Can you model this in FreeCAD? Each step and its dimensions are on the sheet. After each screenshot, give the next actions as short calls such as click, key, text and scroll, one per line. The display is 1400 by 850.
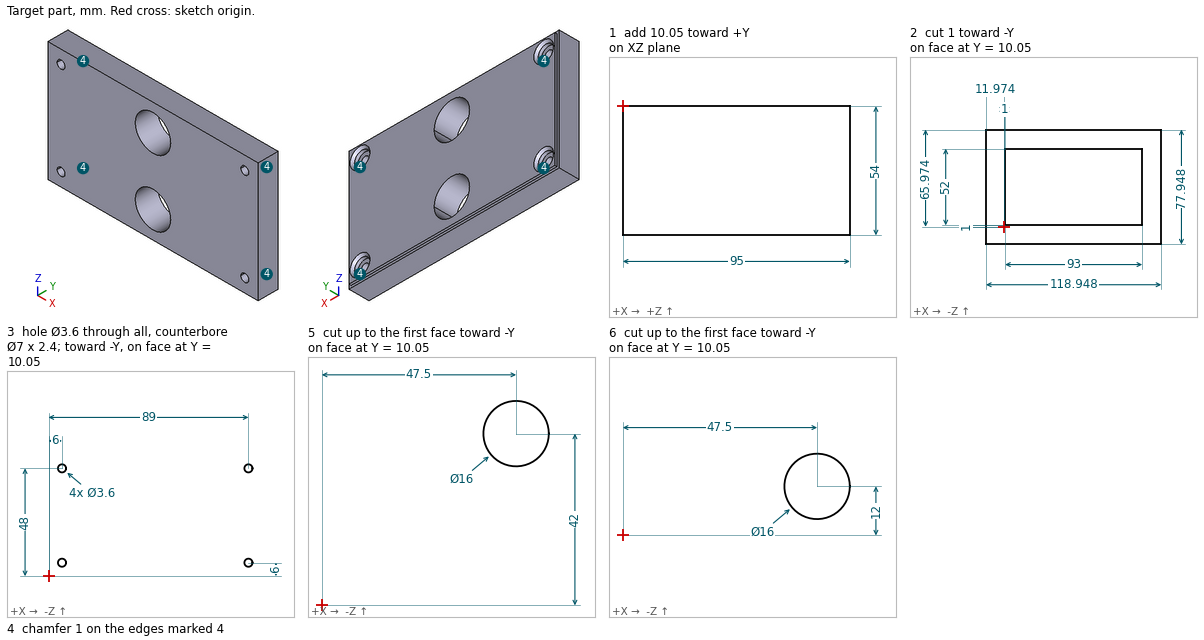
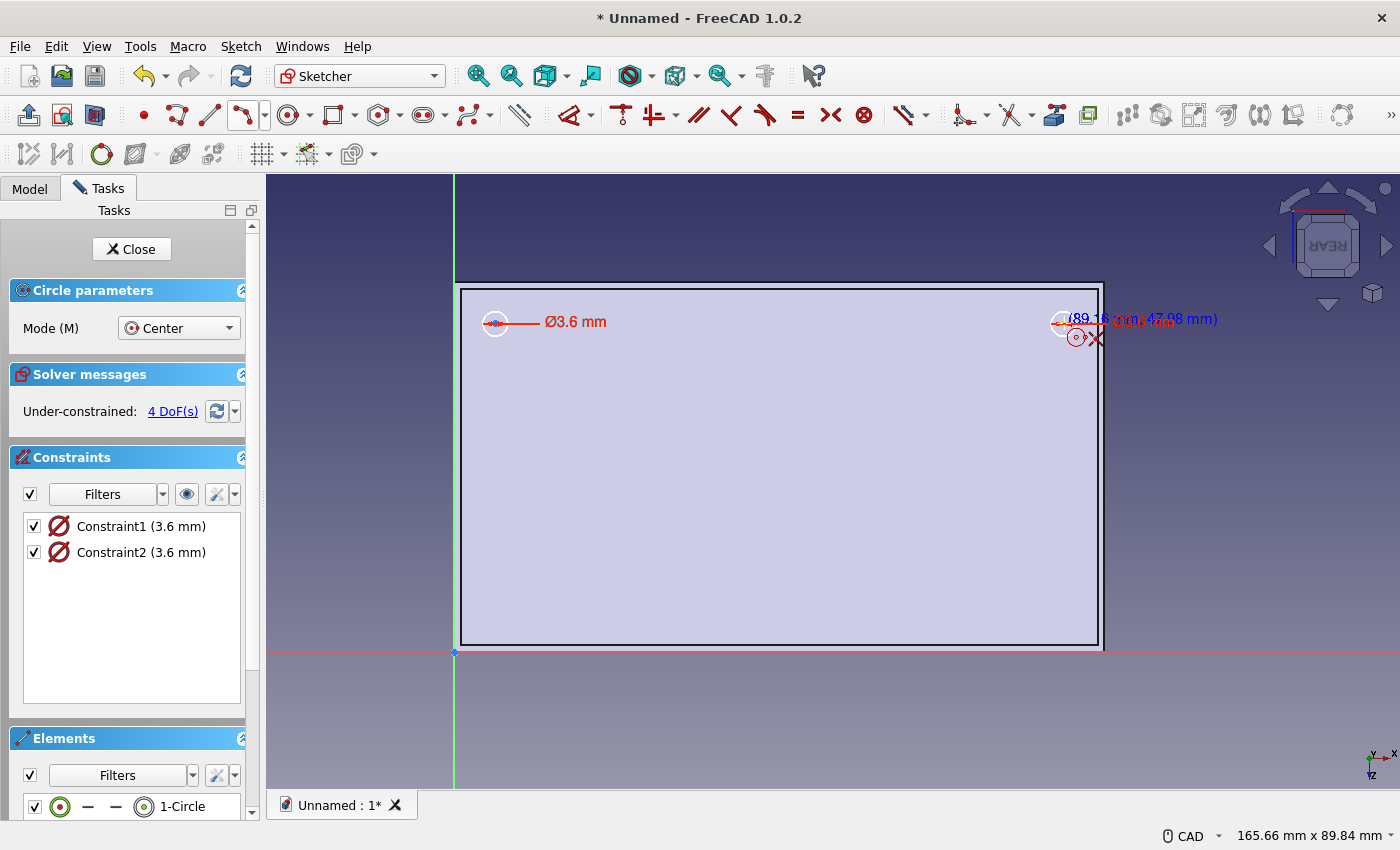
scroll(1063, 611, up, 4)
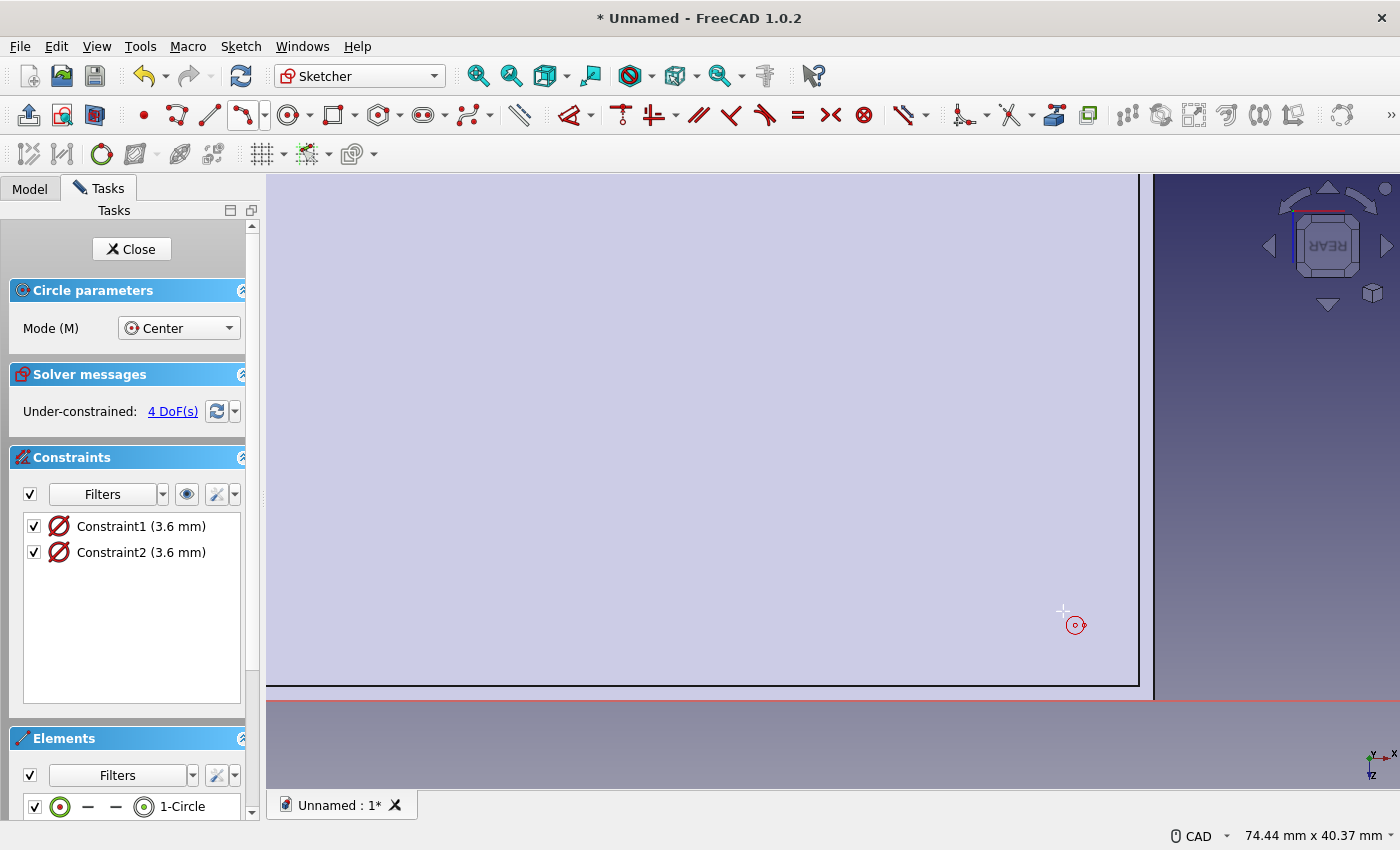
click(1063, 610)
move(1082, 591)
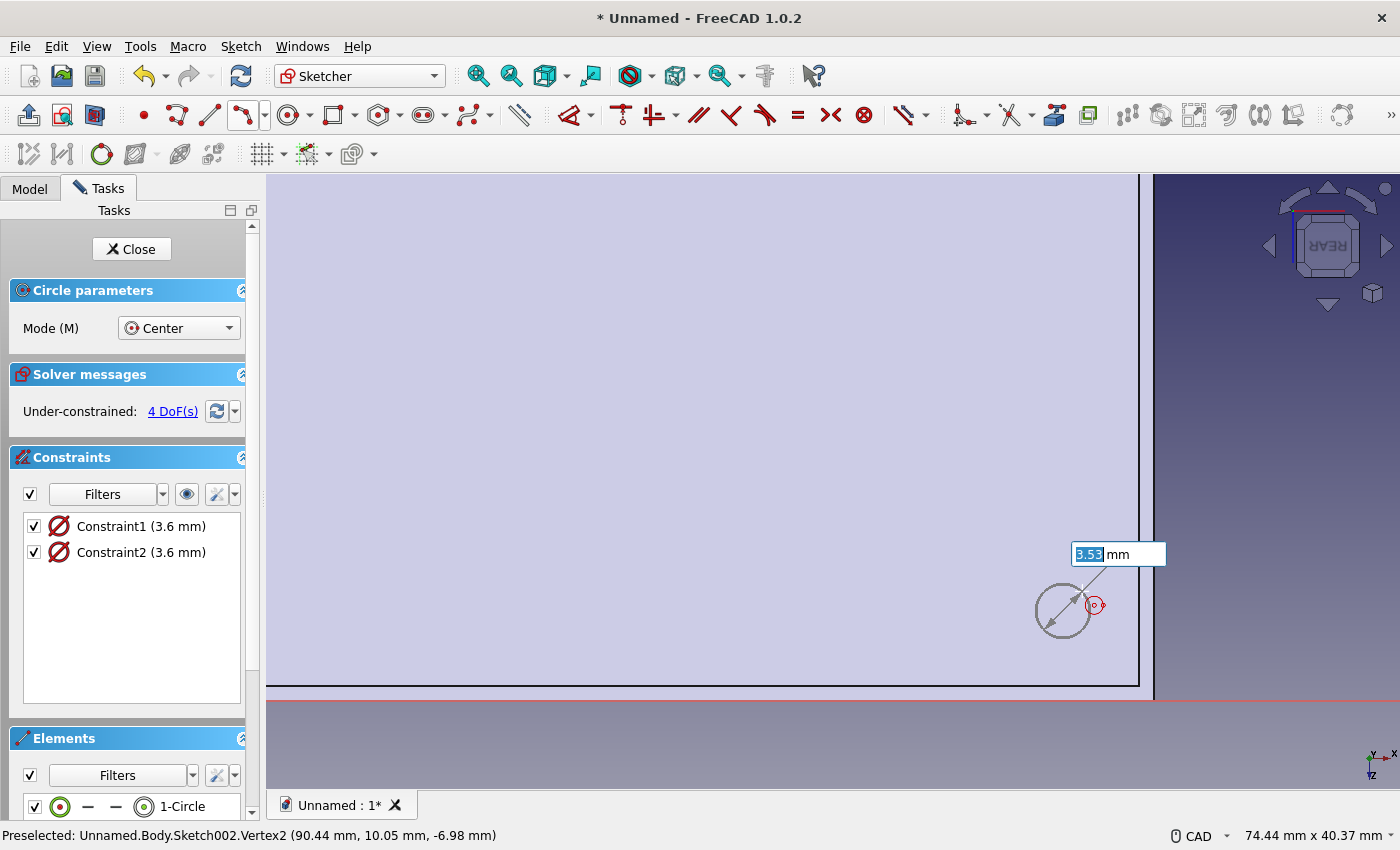
text(3.6)
key(Return)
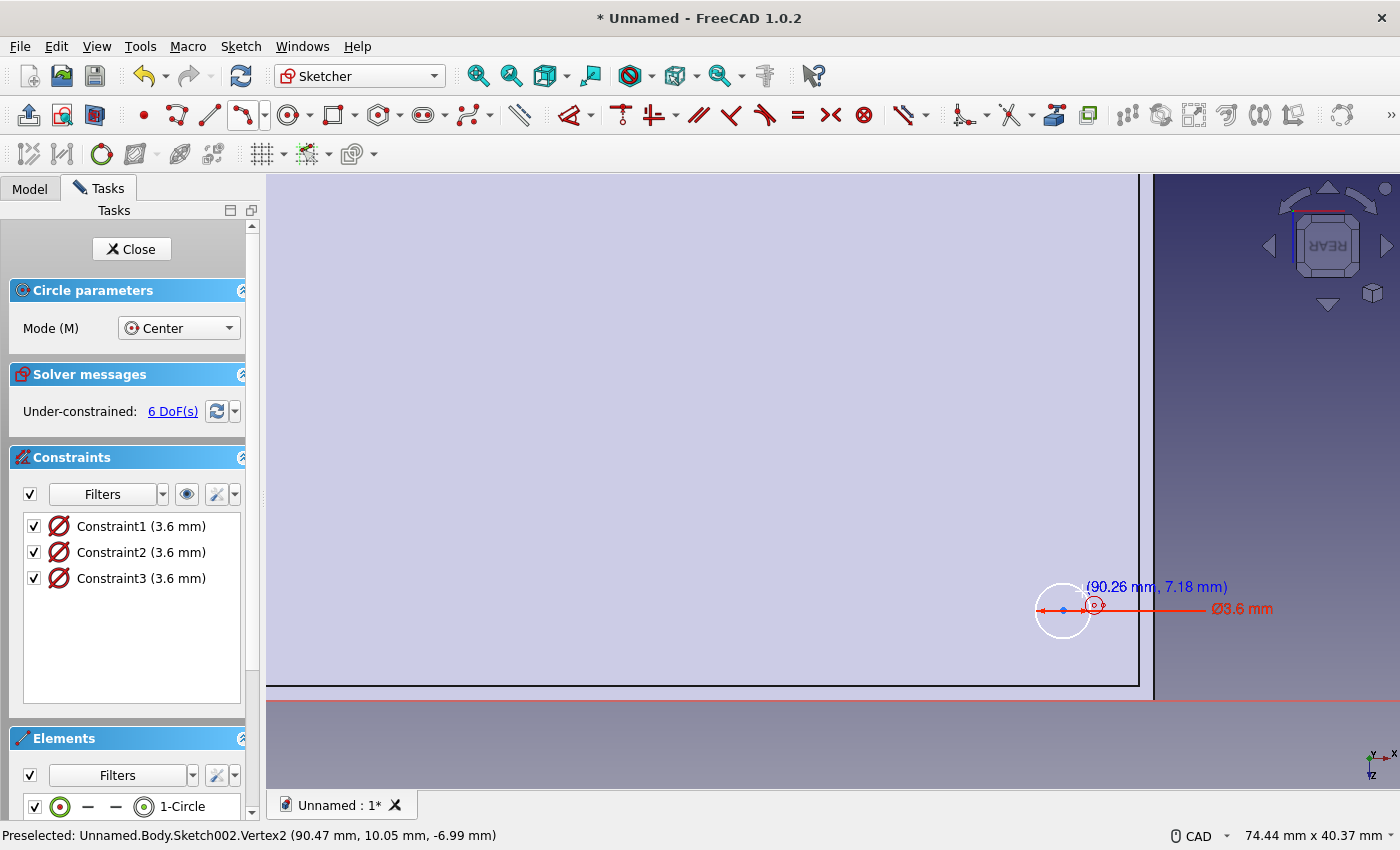
scroll(1063, 612, down, 4)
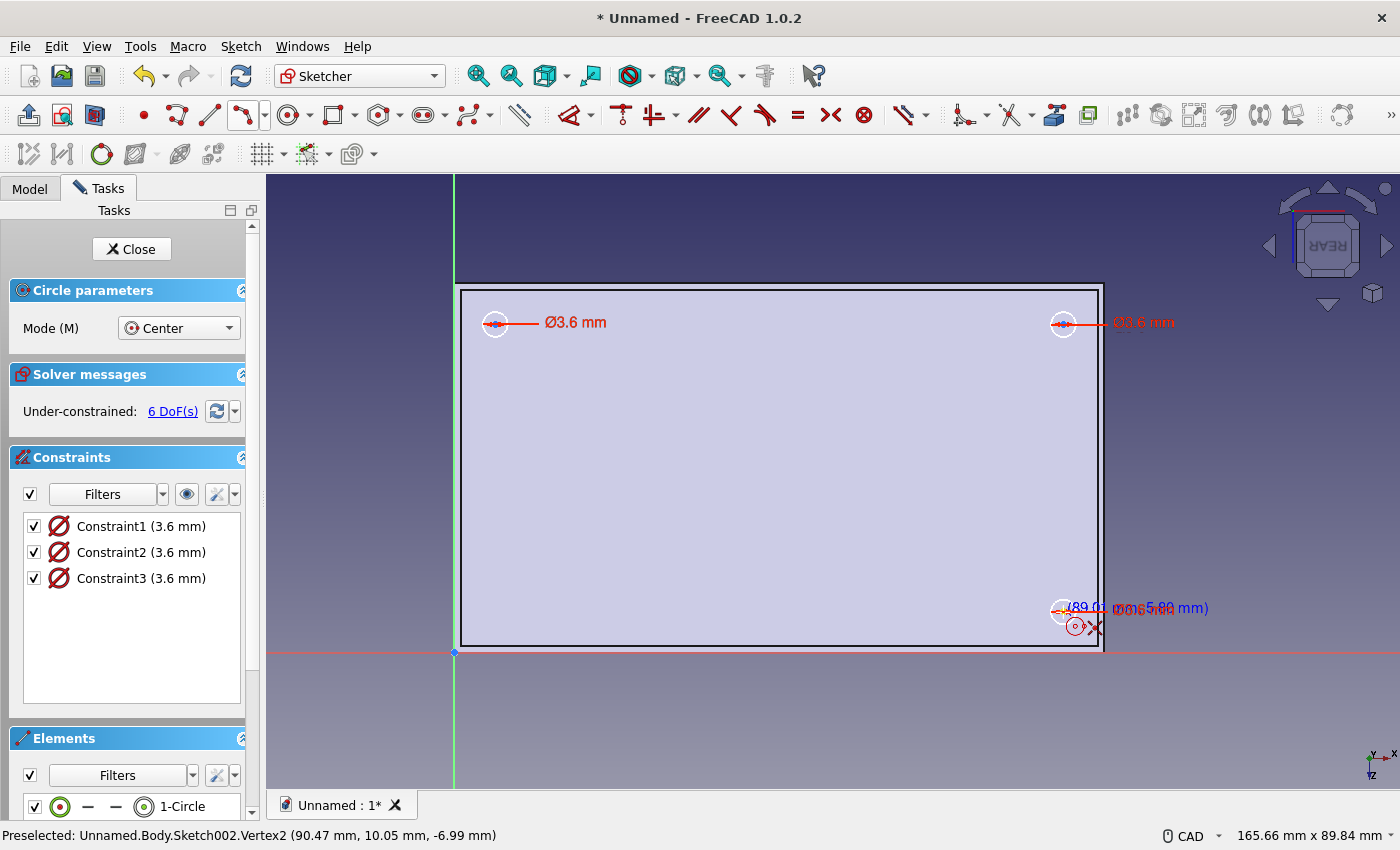
scroll(495, 611, up, 4)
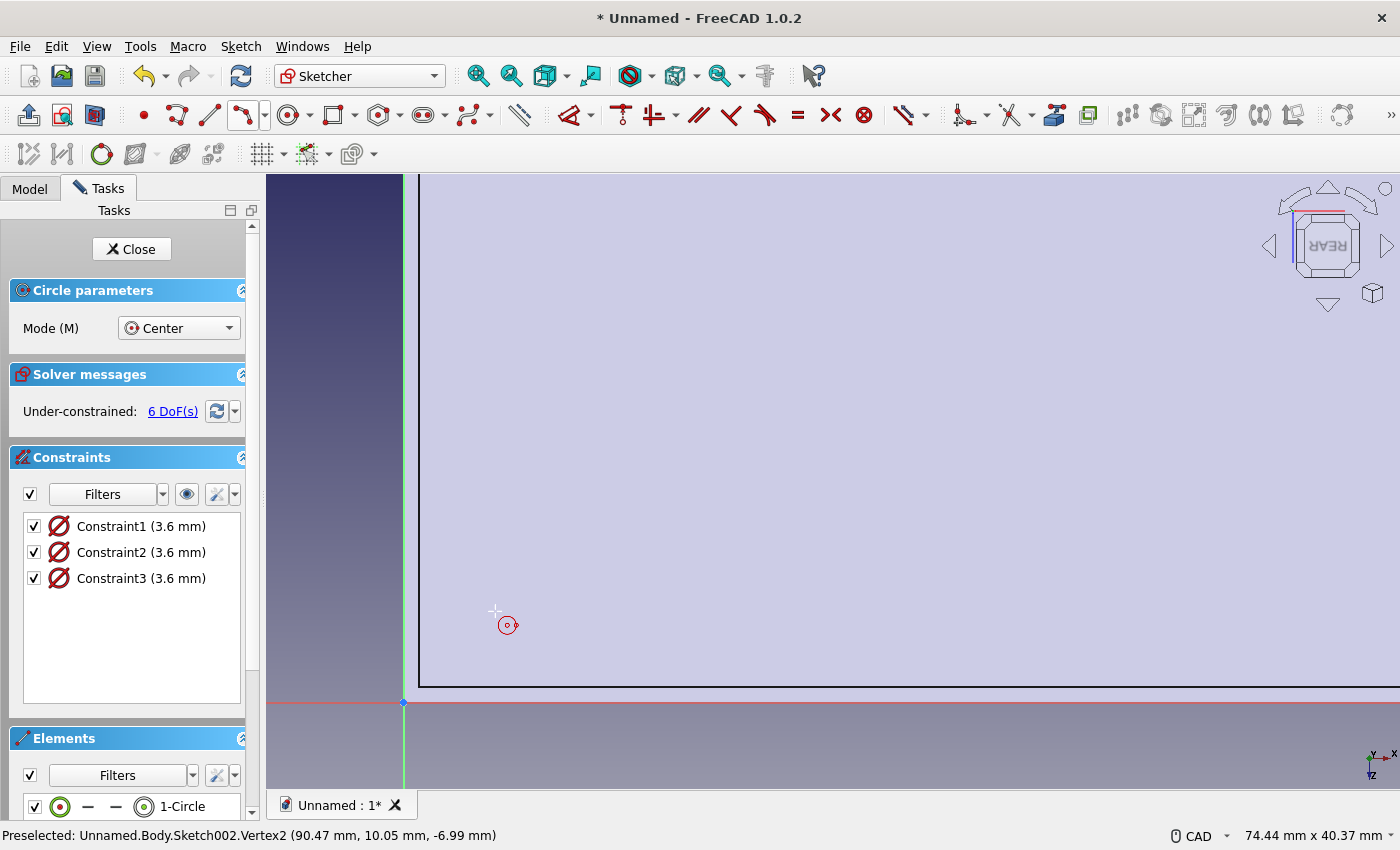
click(495, 611)
move(515, 592)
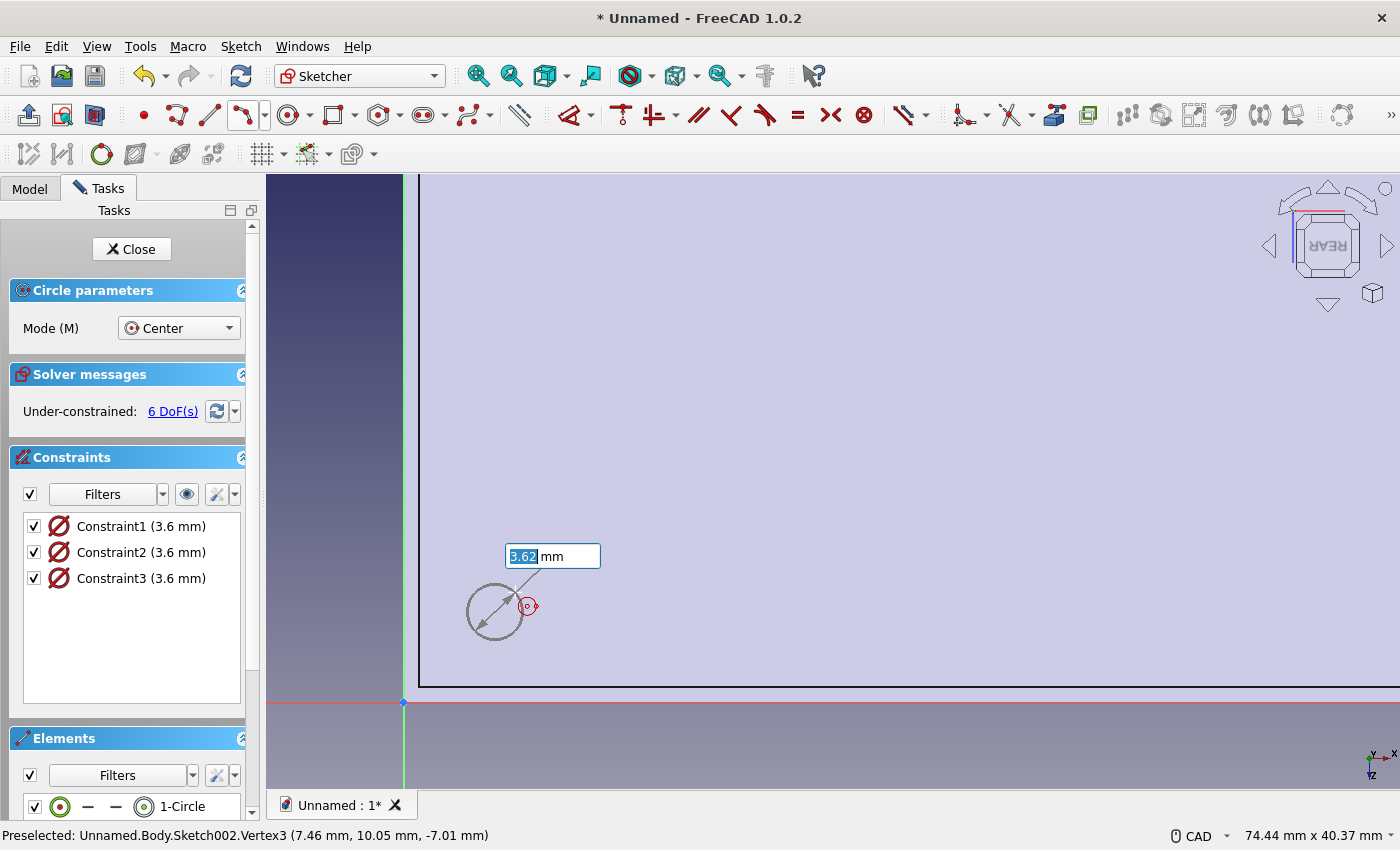
text(3.6)
key(Return)
key(Escape)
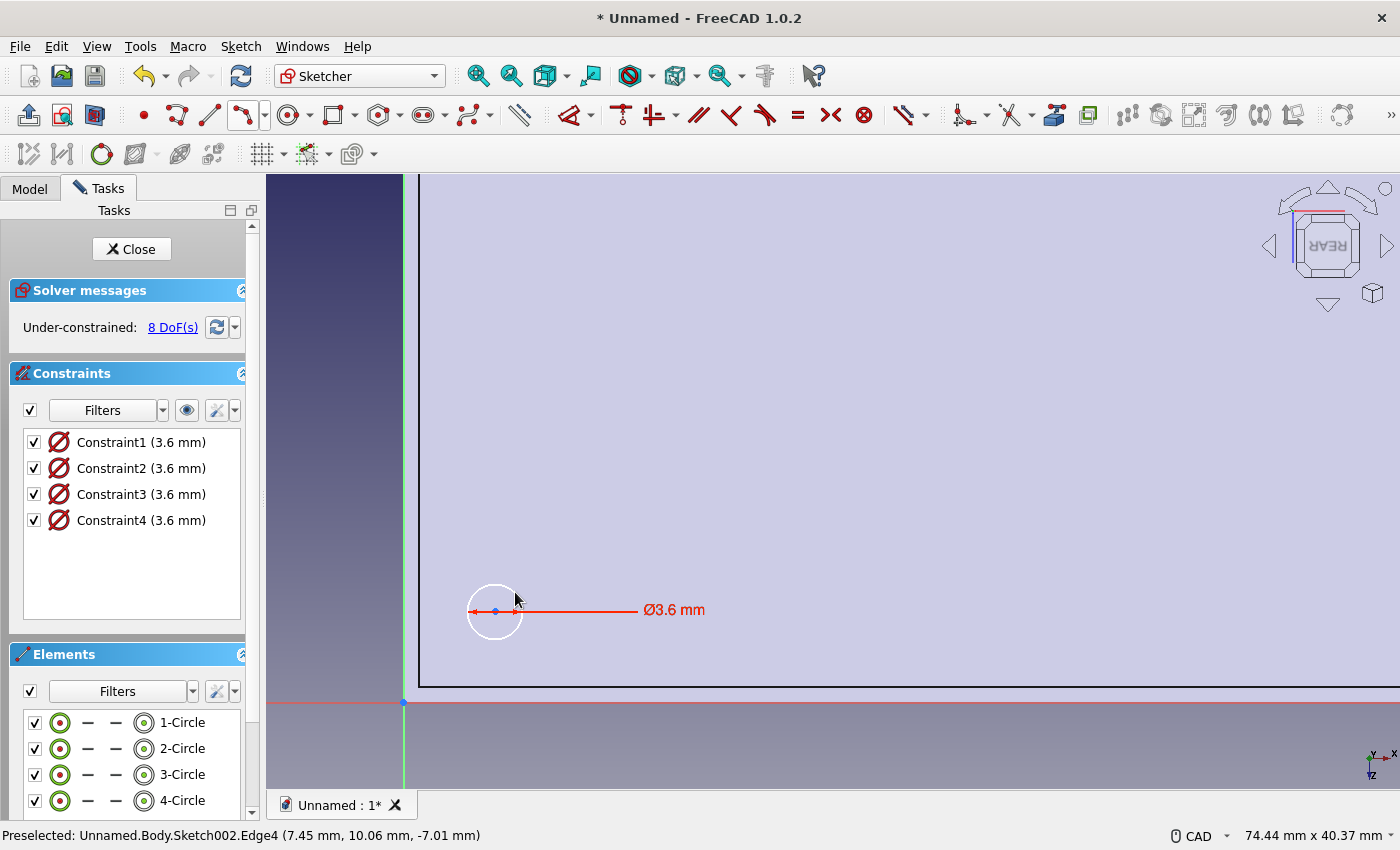
scroll(495, 611, down, 4)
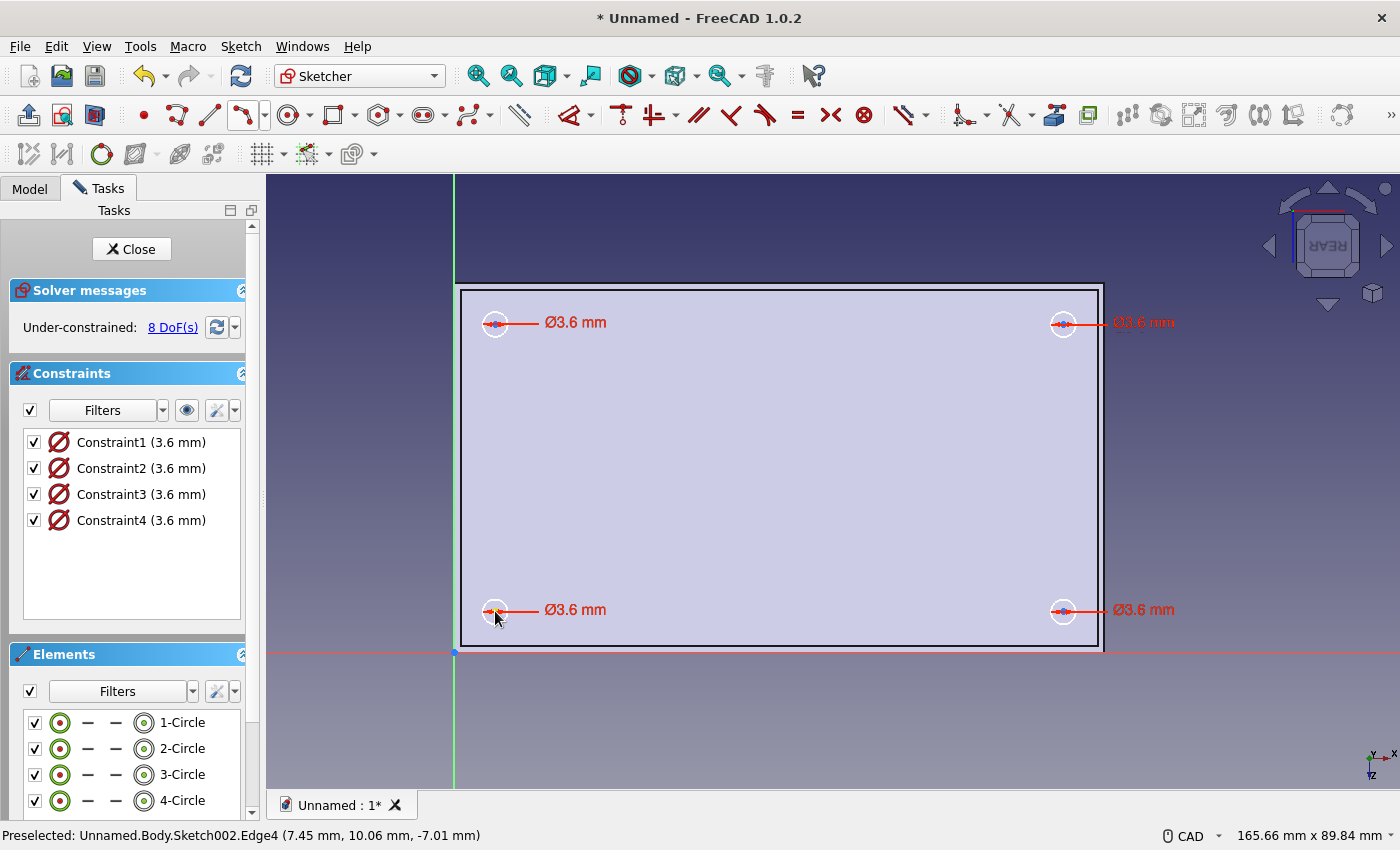
click(495, 324)